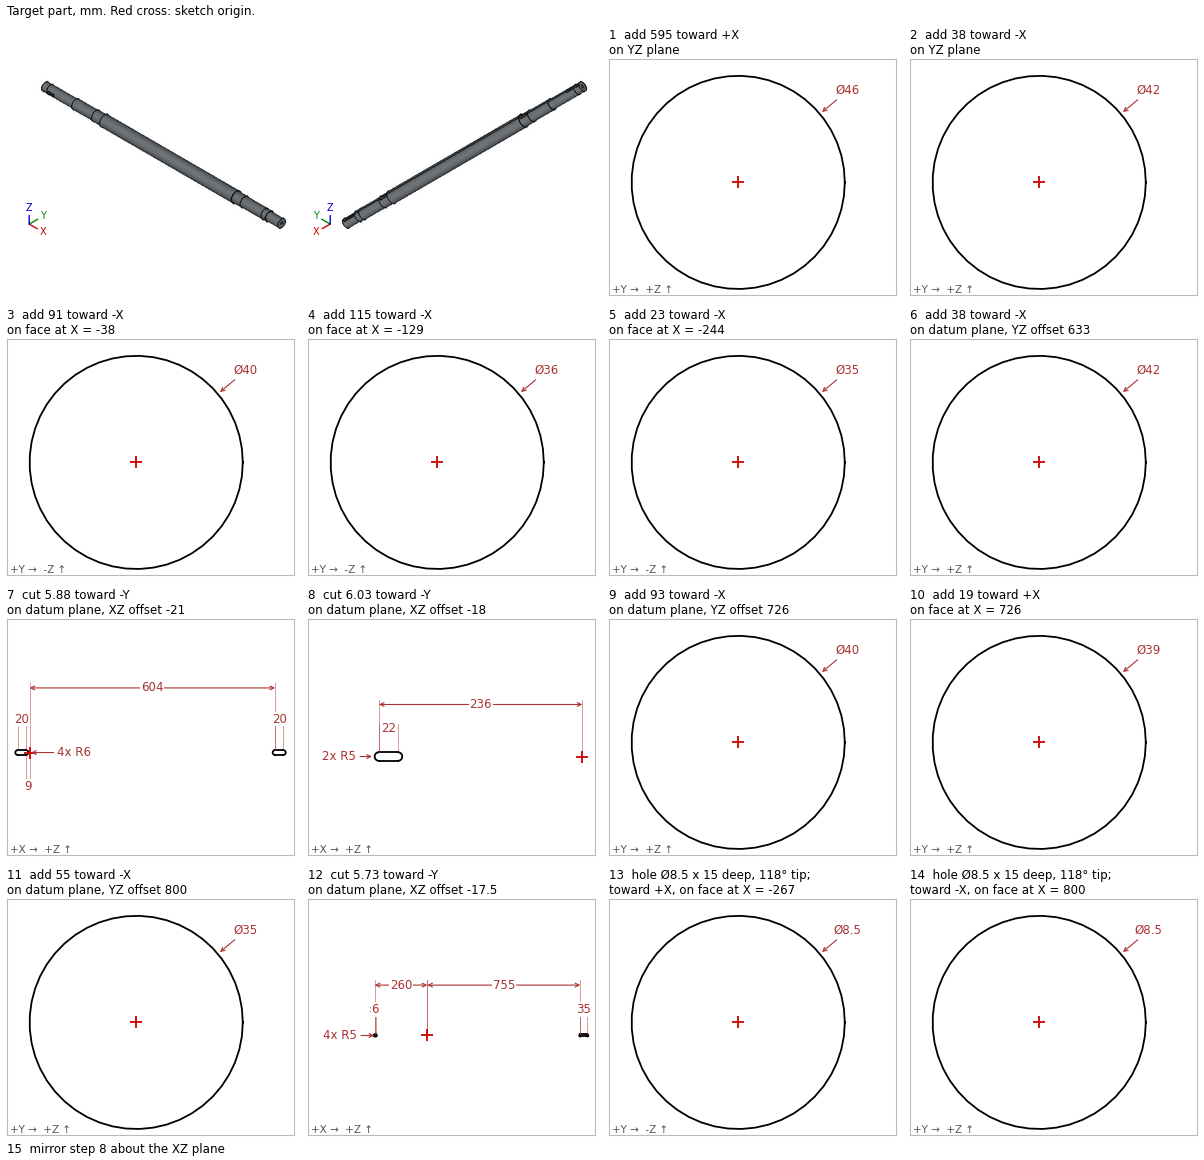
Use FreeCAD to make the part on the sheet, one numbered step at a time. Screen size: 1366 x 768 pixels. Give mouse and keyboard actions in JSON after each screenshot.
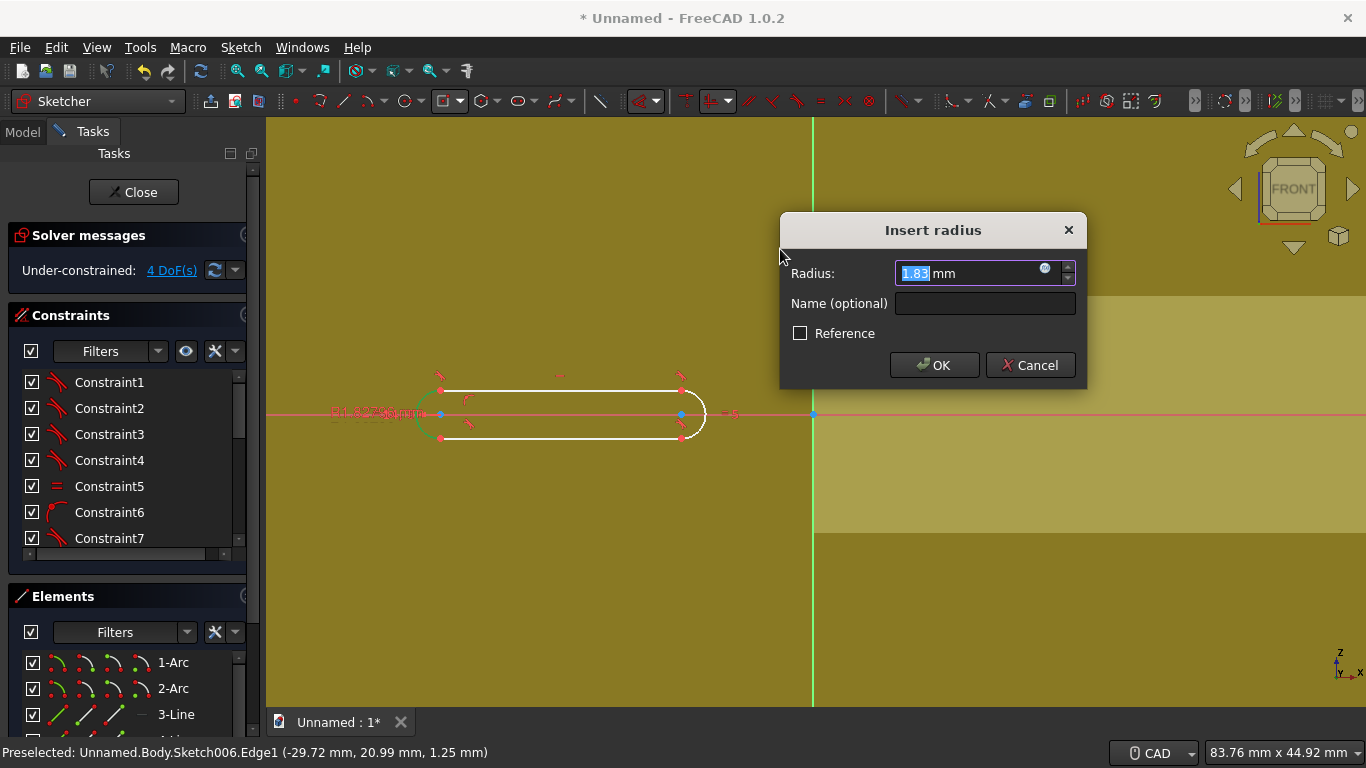
{"action": "type", "text": "6"}
{"action": "key", "text": "Return"}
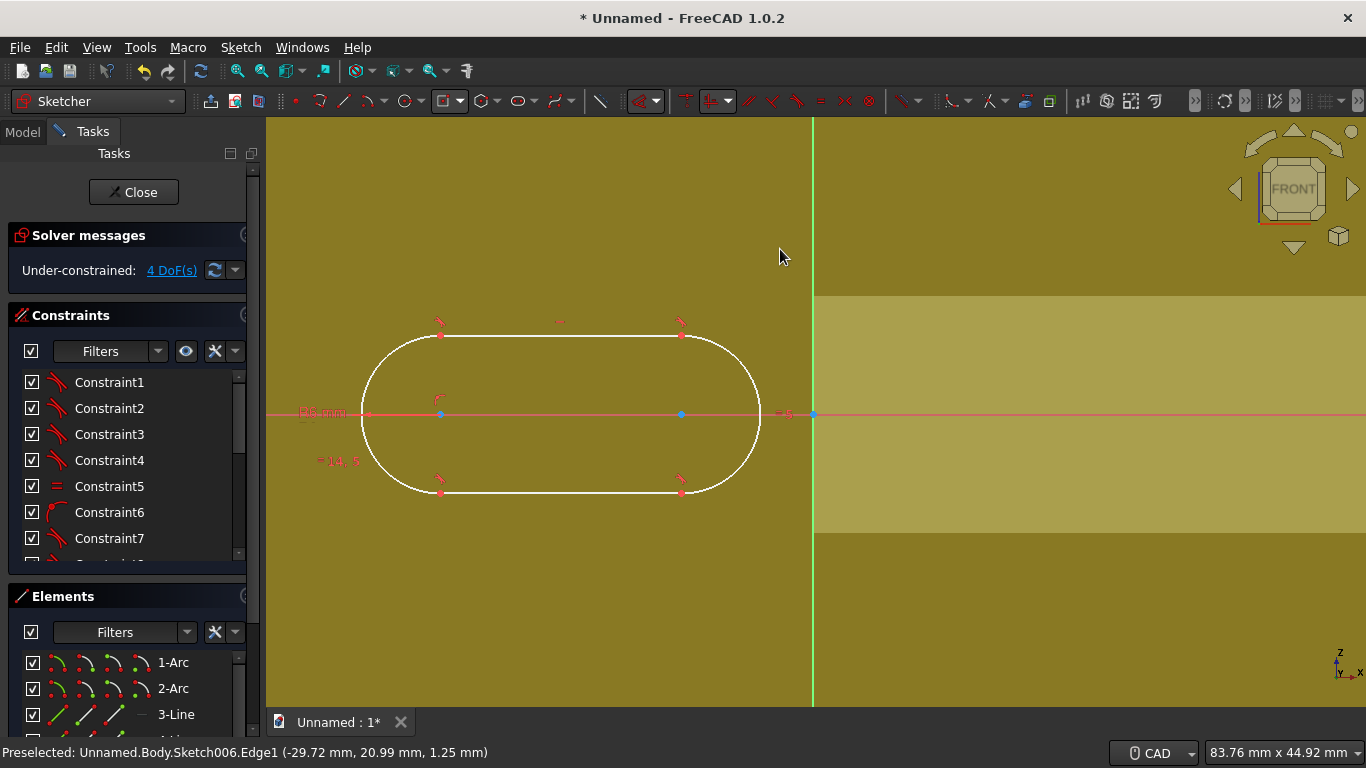
{"action": "scroll", "coordinate": [429, 412], "scroll_direction": "down", "scroll_amount": 13}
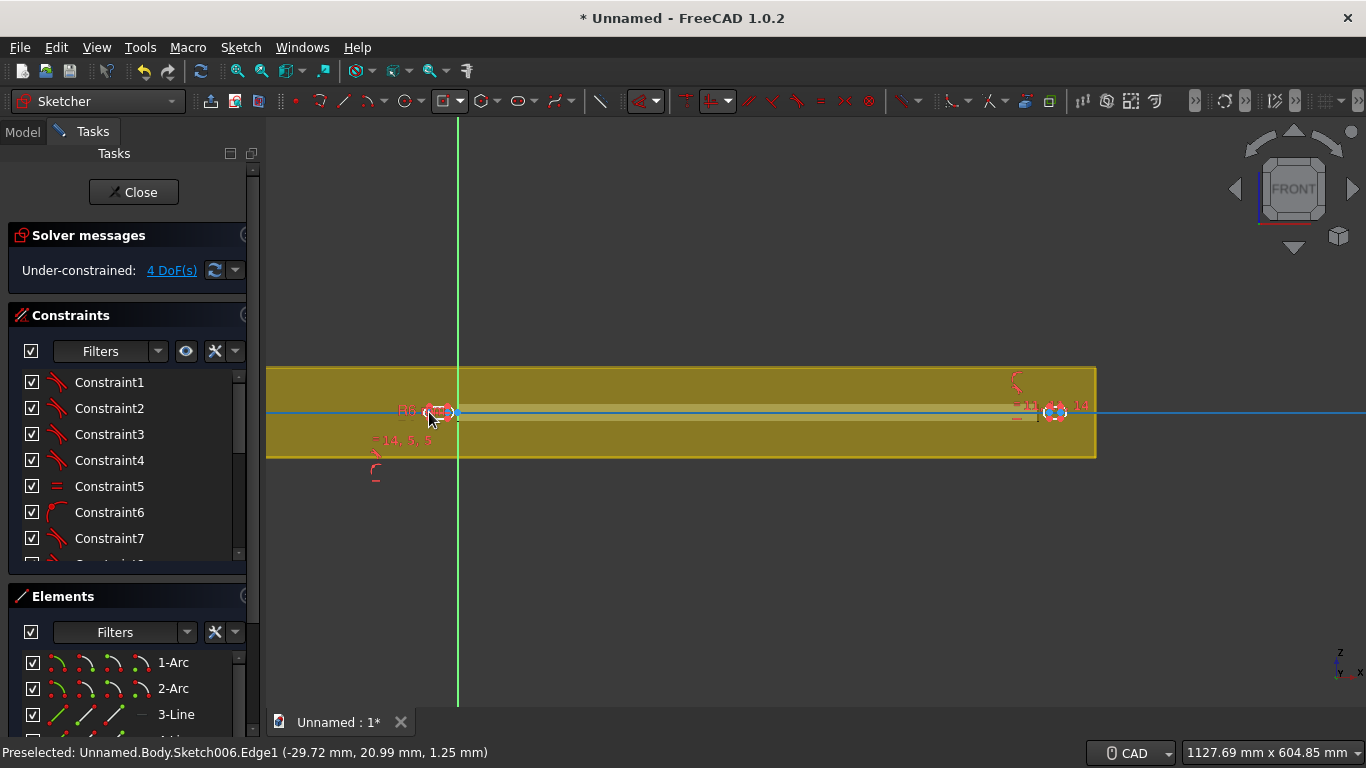
{"action": "scroll", "coordinate": [435, 407], "scroll_direction": "up", "scroll_amount": 5}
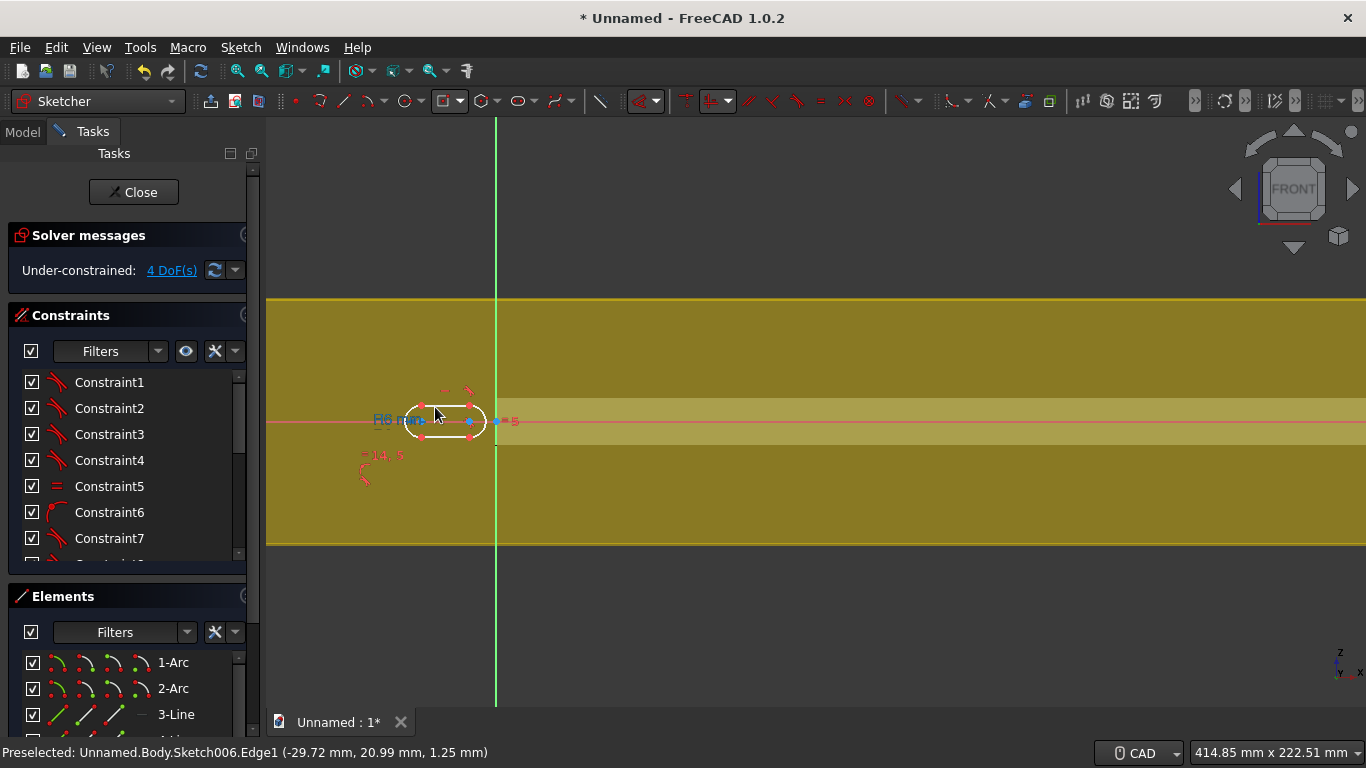
{"action": "left_click", "coordinate": [436, 406]}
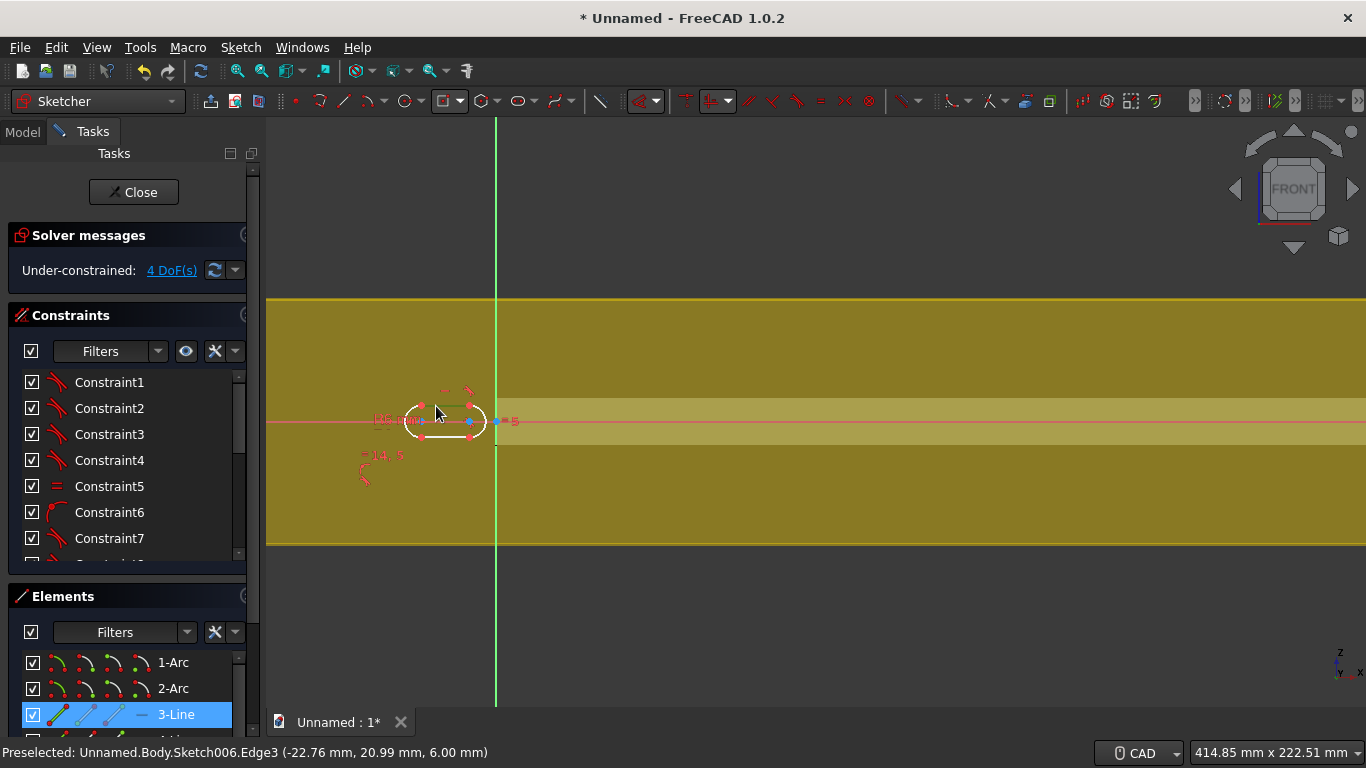
{"action": "left_click", "coordinate": [658, 102]}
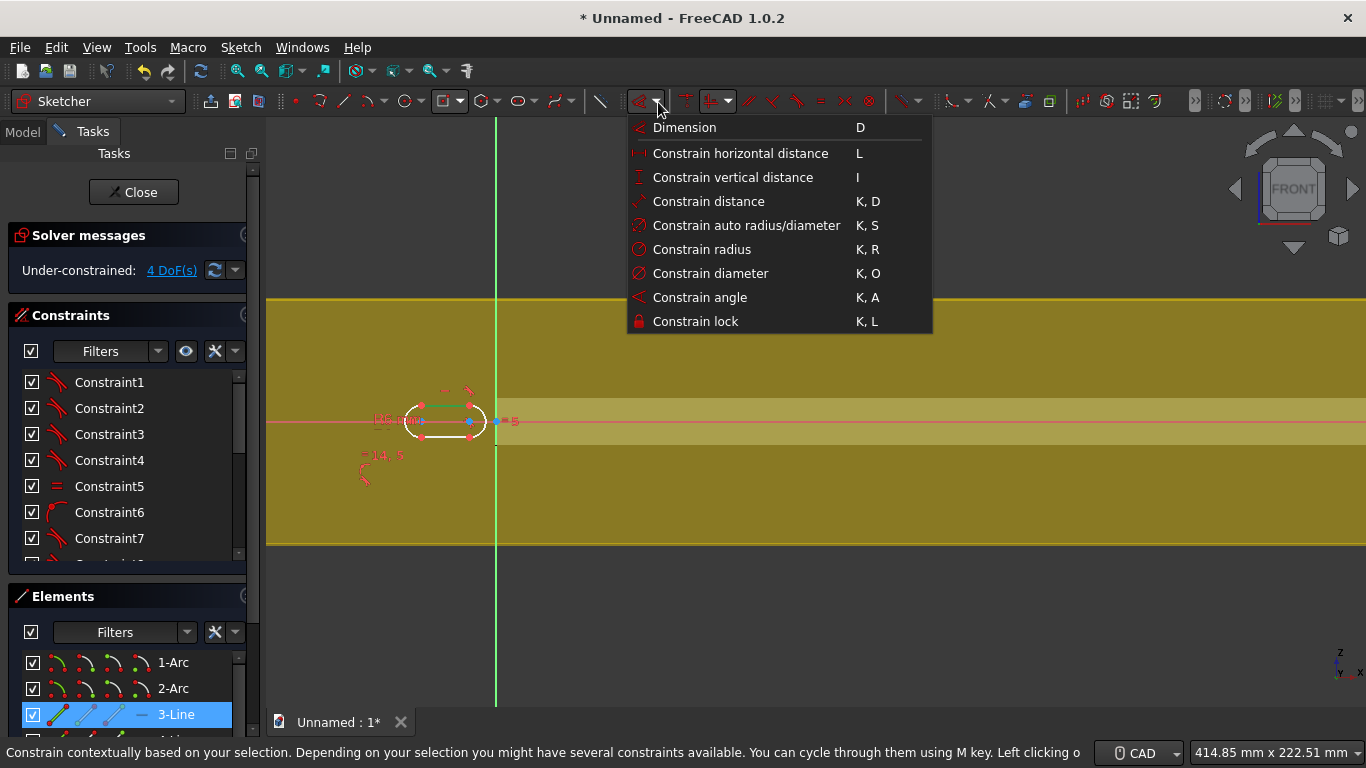
{"action": "left_click", "coordinate": [780, 153]}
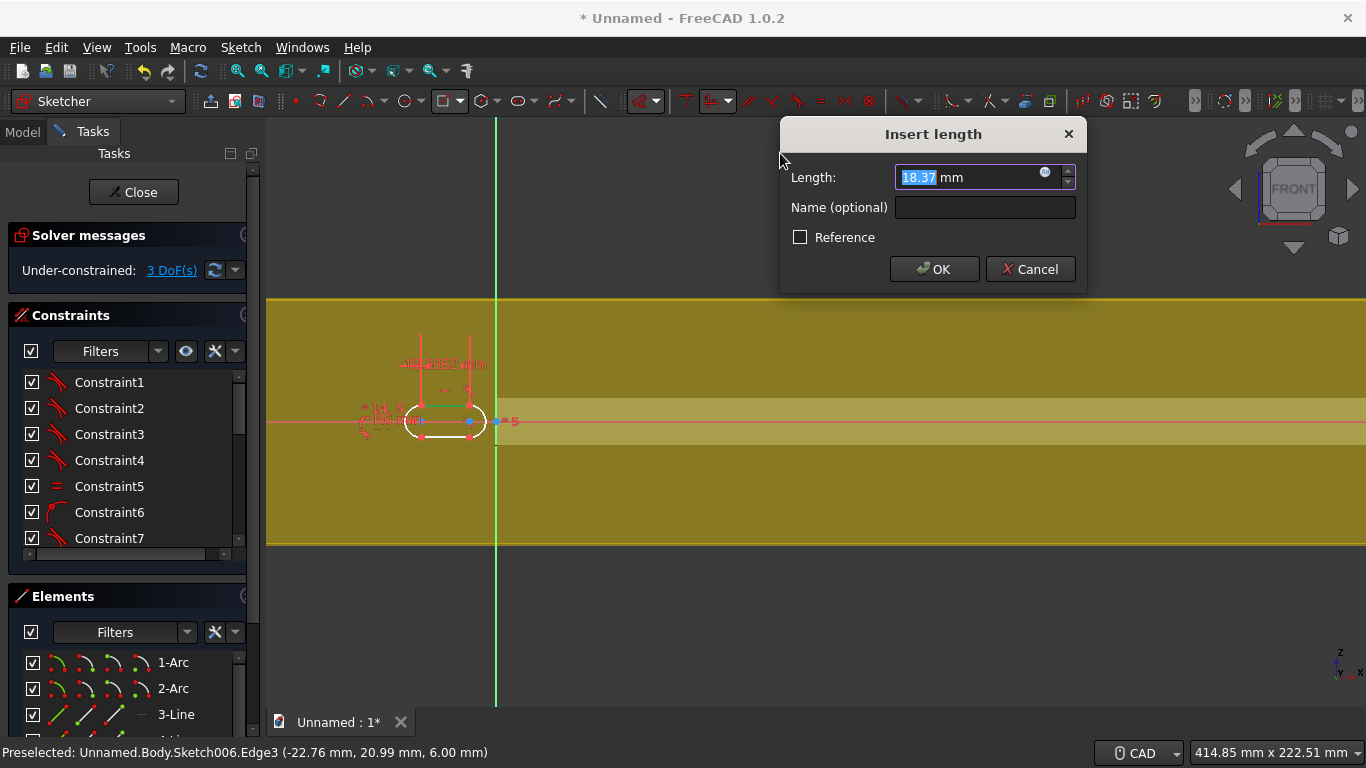
{"action": "type", "text": "20"}
{"action": "key", "text": "Return"}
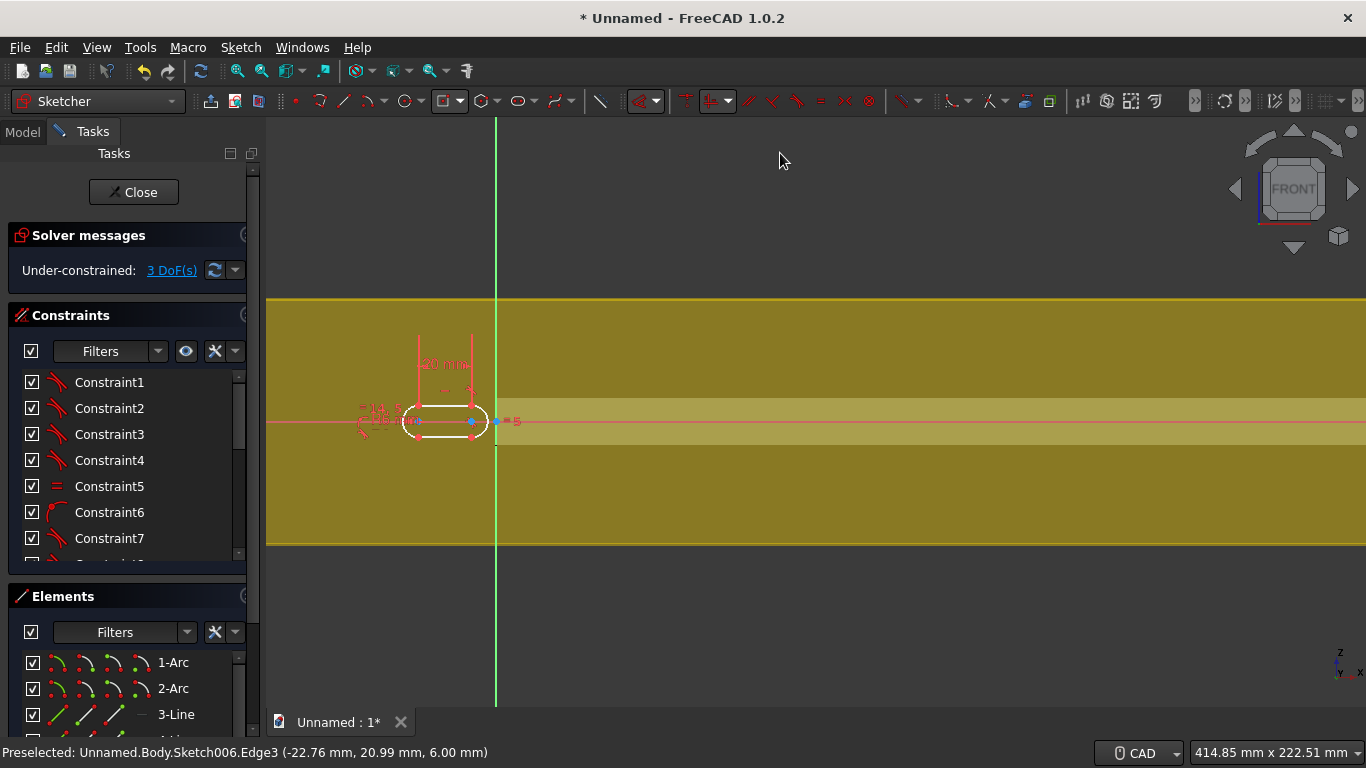
{"action": "scroll", "coordinate": [435, 406], "scroll_direction": "down", "scroll_amount": 5}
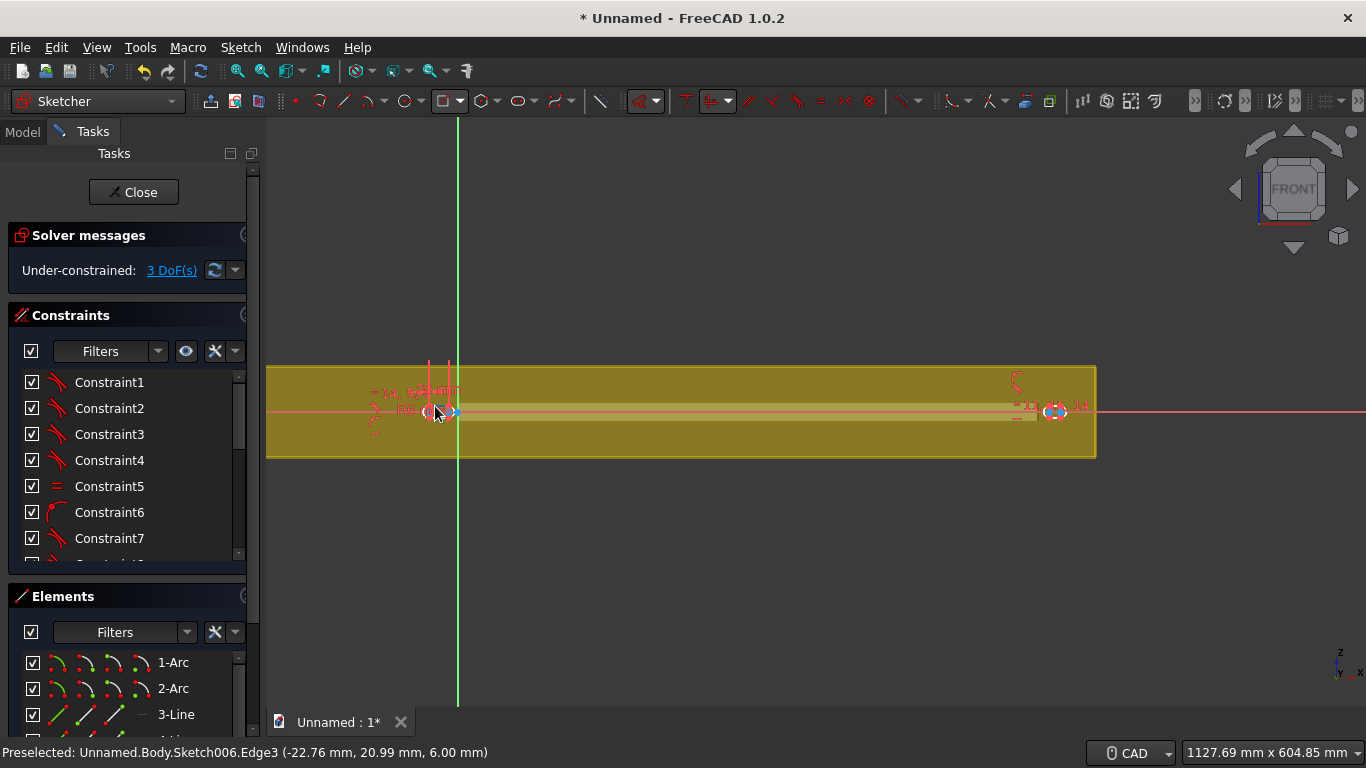
{"action": "scroll", "coordinate": [1053, 406], "scroll_direction": "up", "scroll_amount": 8}